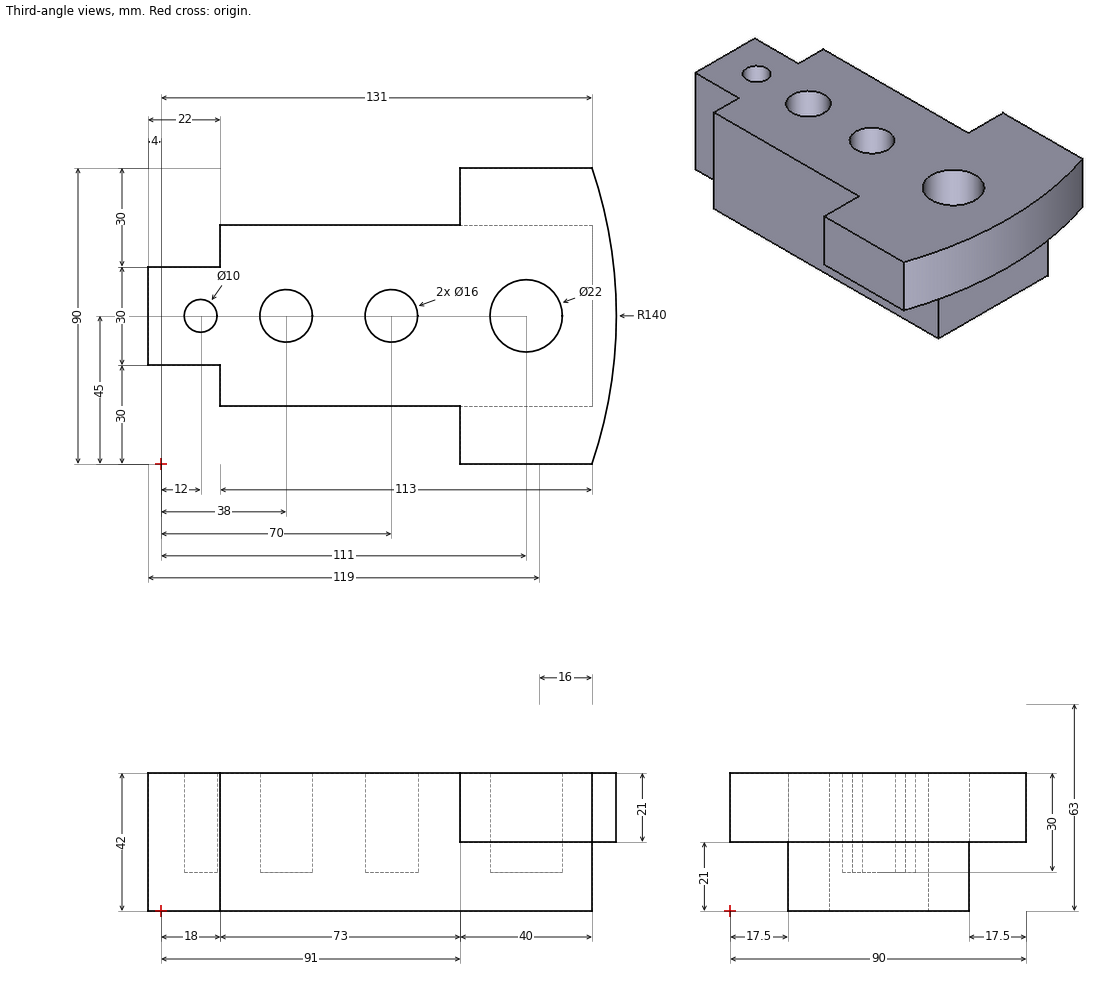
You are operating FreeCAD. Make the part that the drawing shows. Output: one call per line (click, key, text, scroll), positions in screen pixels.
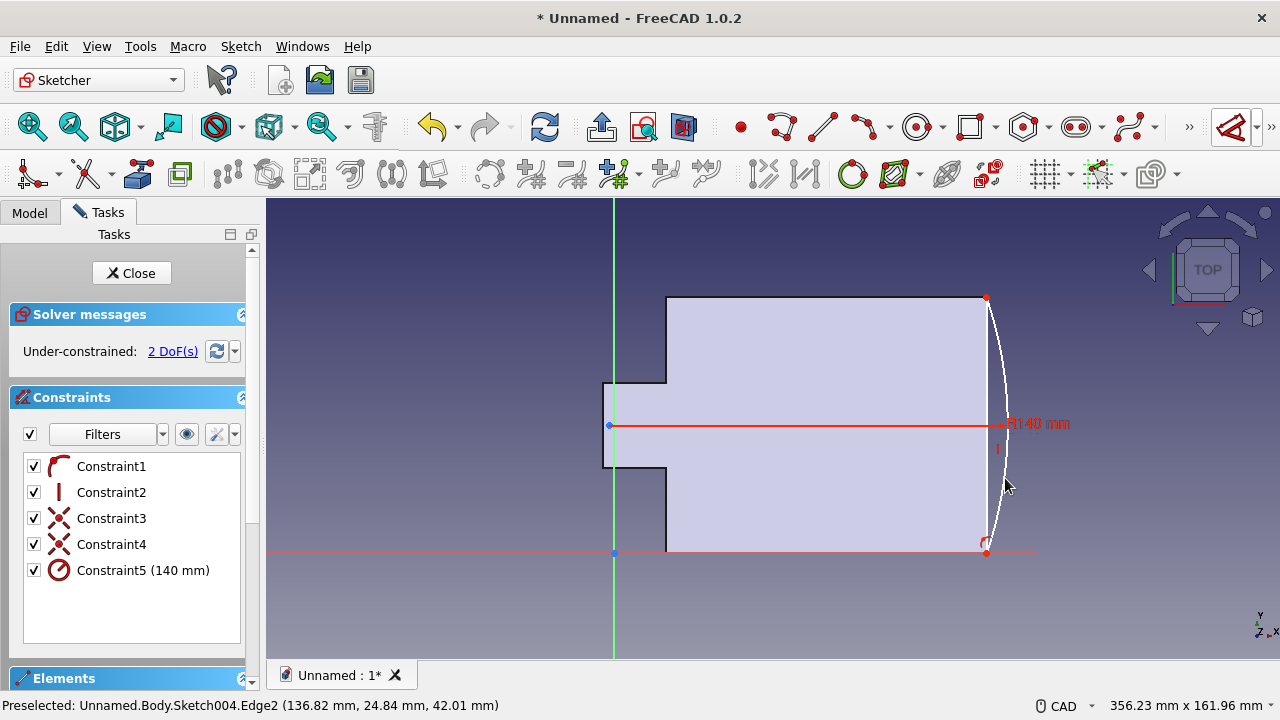
click(987, 375)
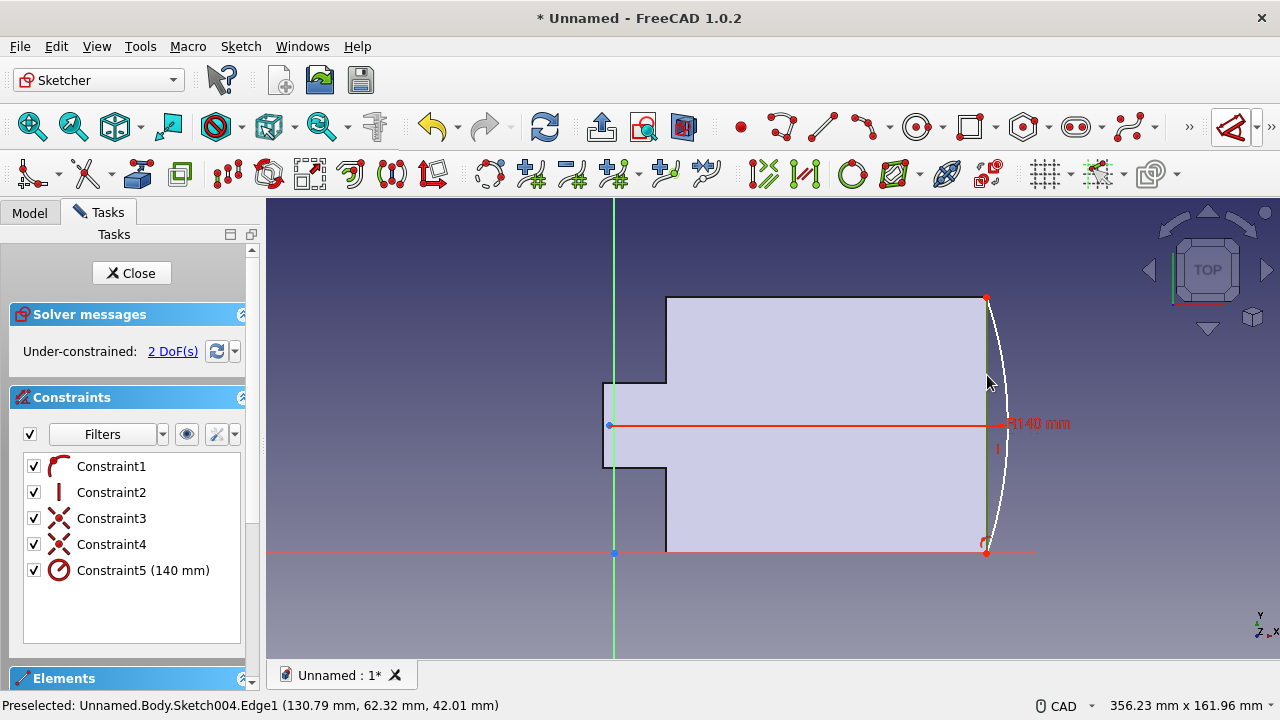
key(i)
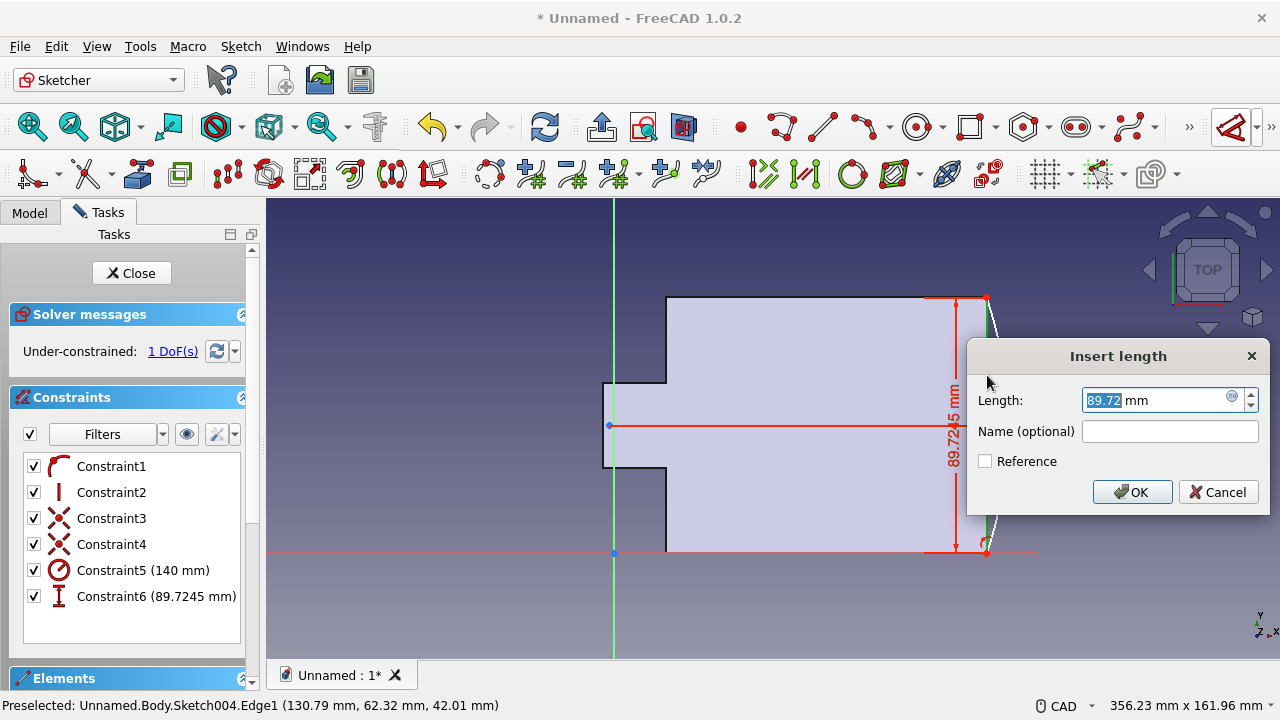
text(90)
key(Return)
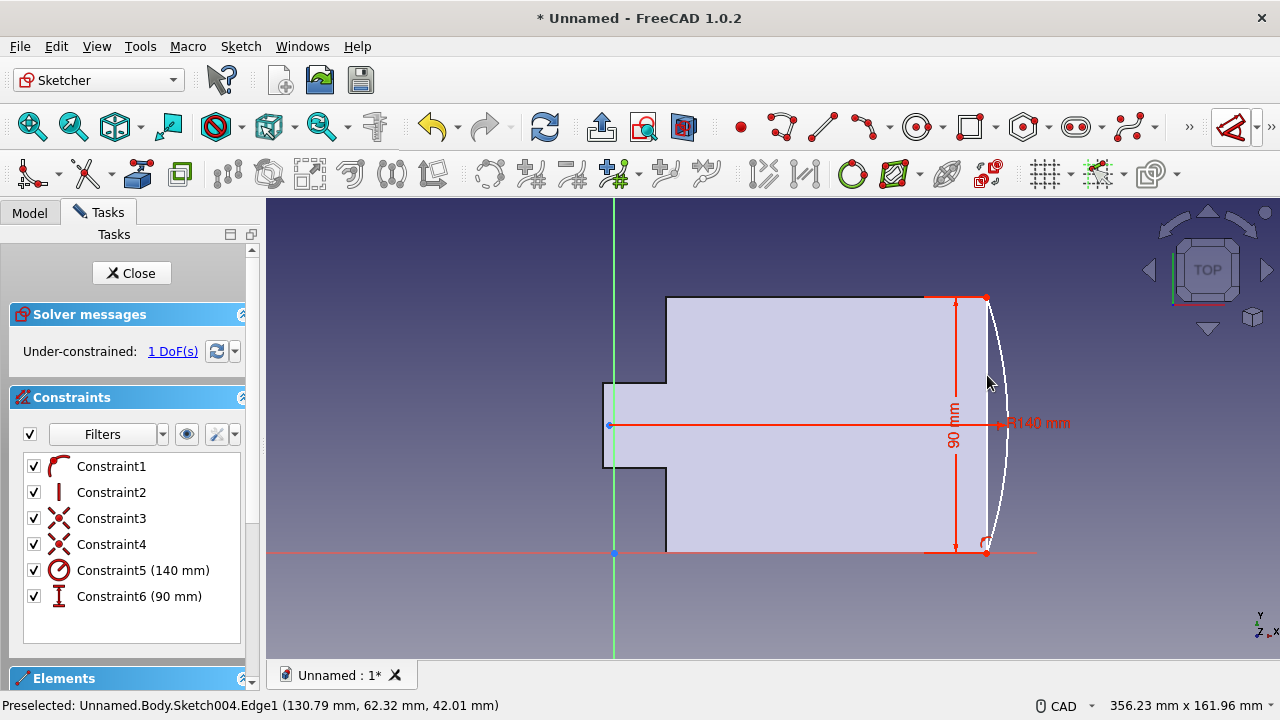
click(987, 297)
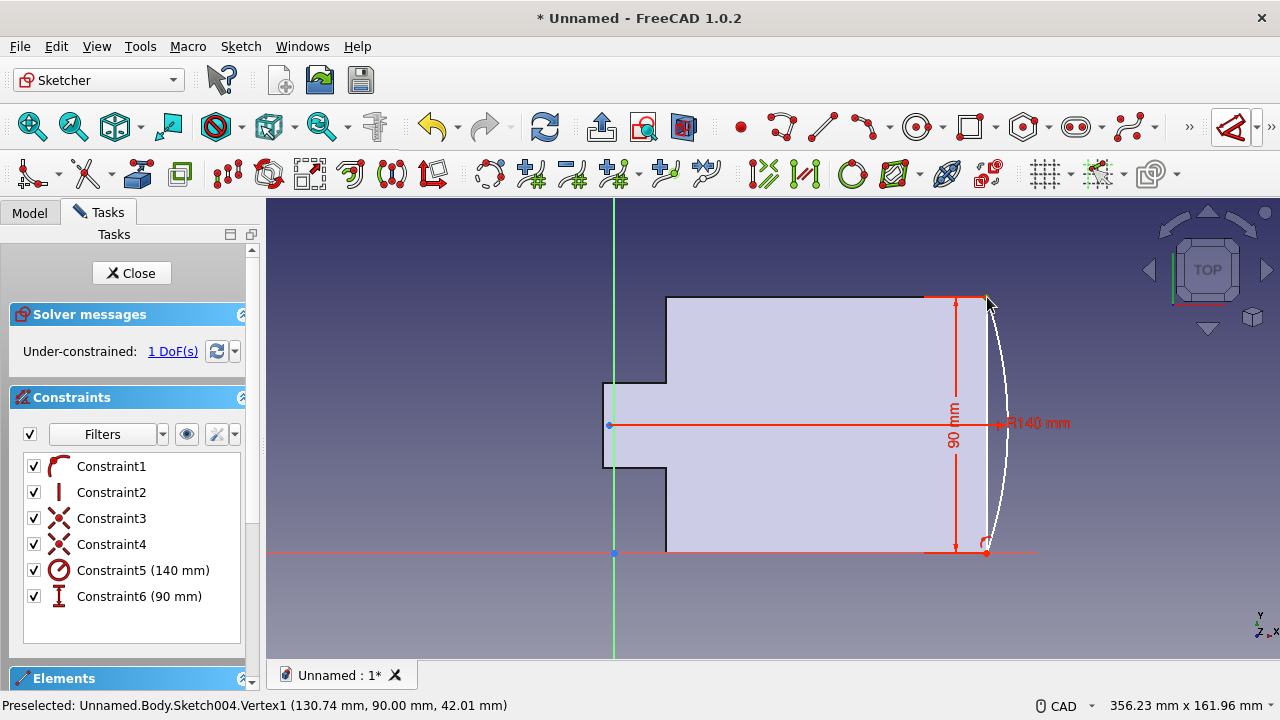
click(1256, 128)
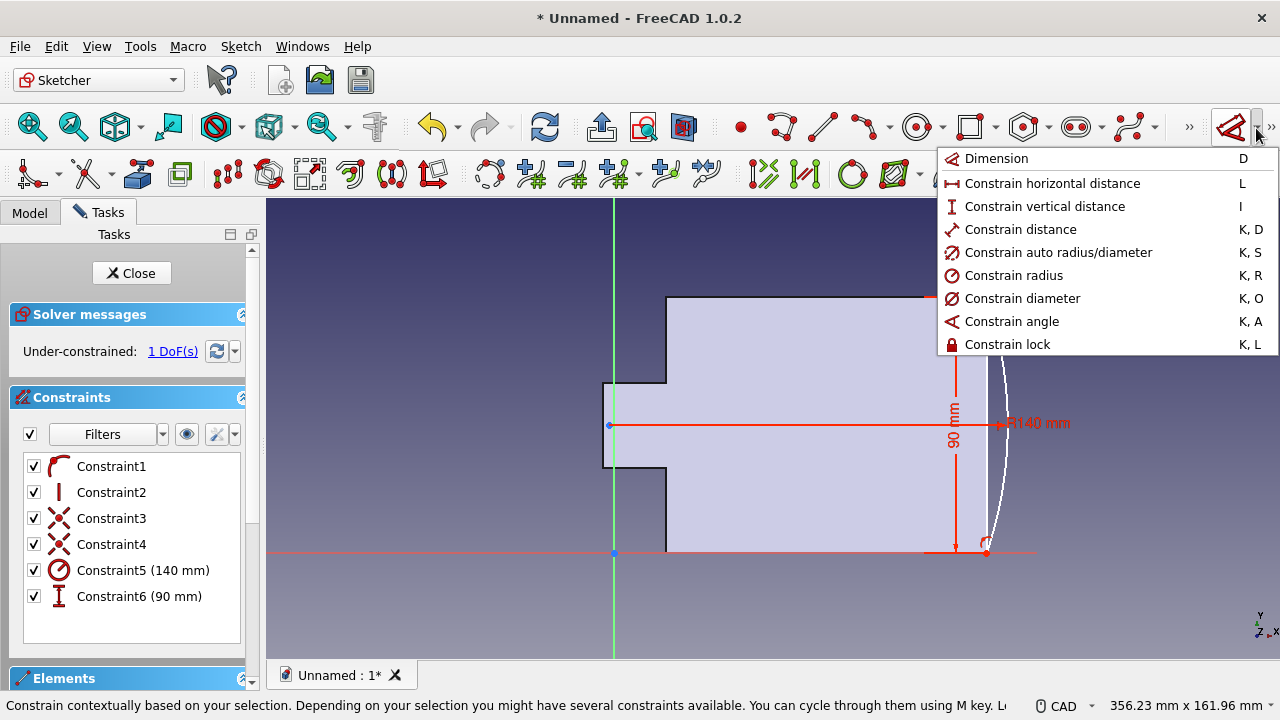
click(1108, 184)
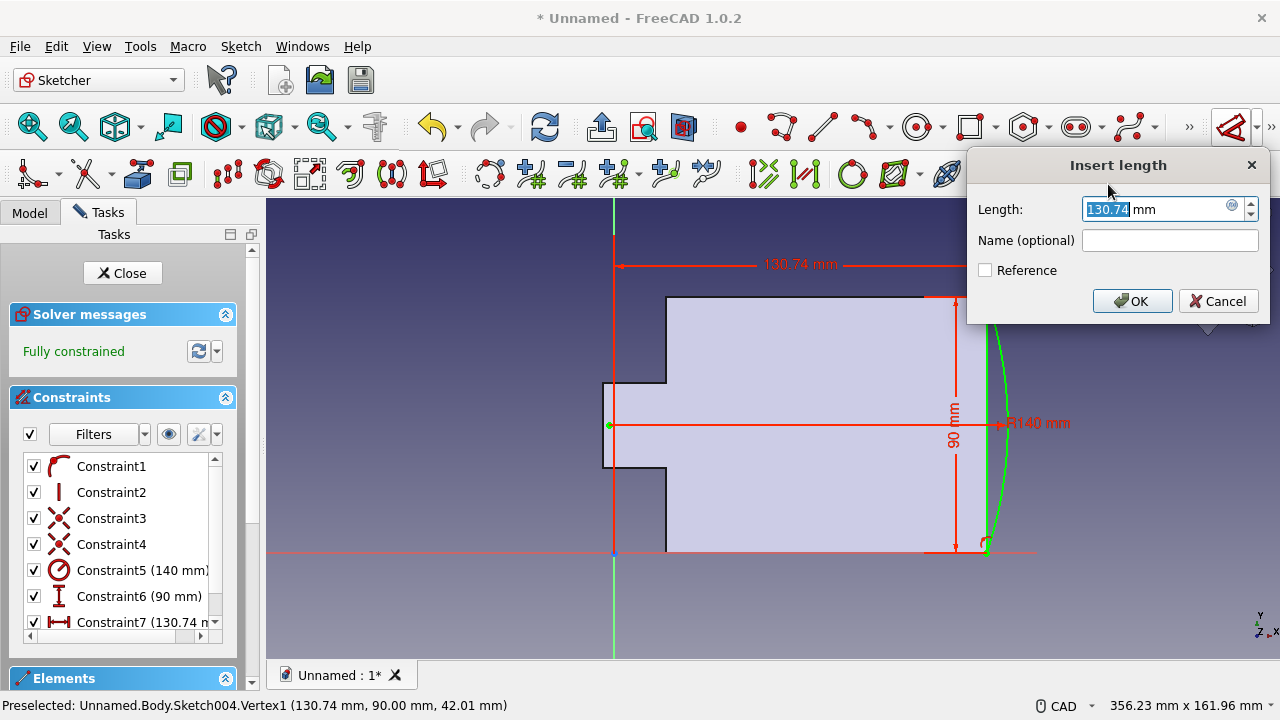
text(131)
key(Return)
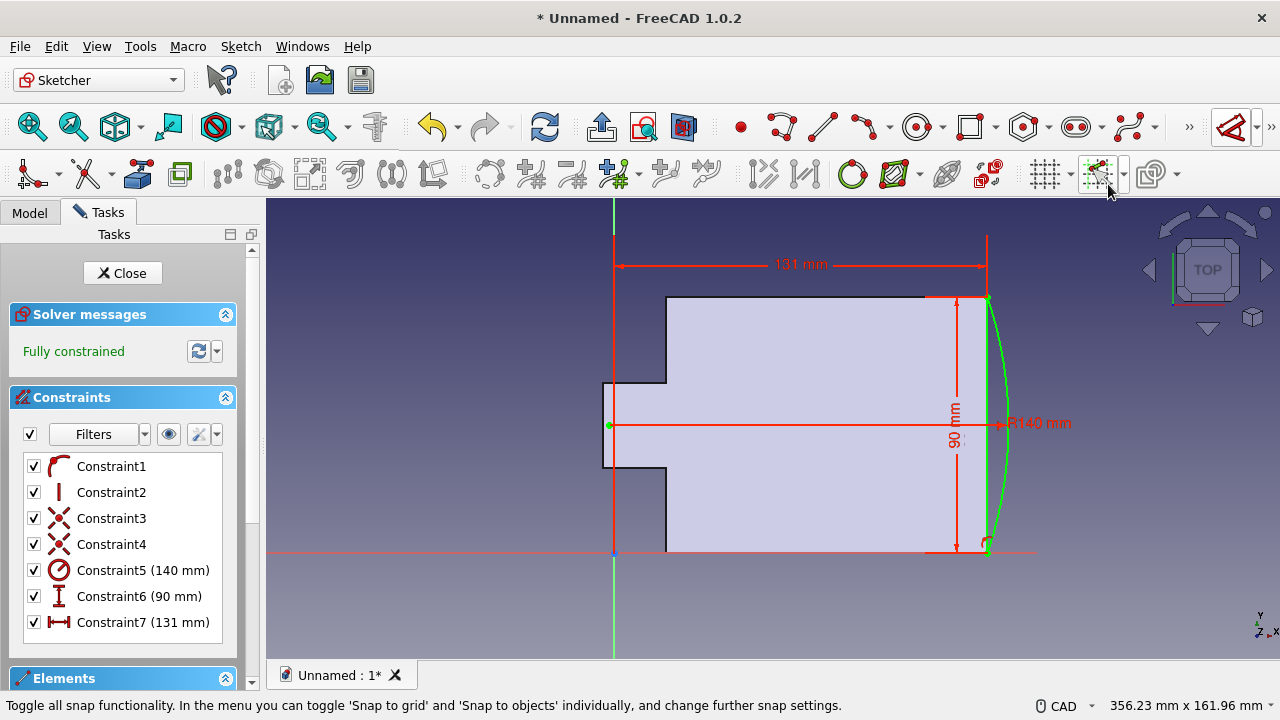
click(123, 273)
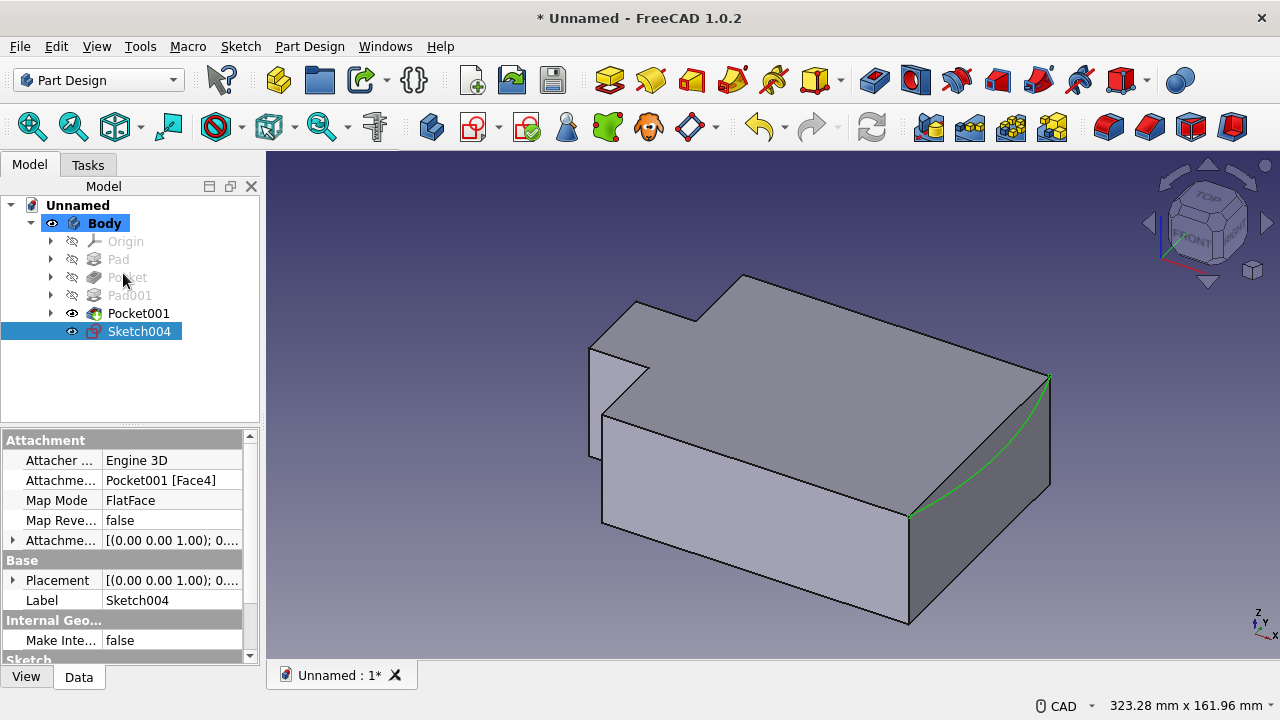
click(610, 80)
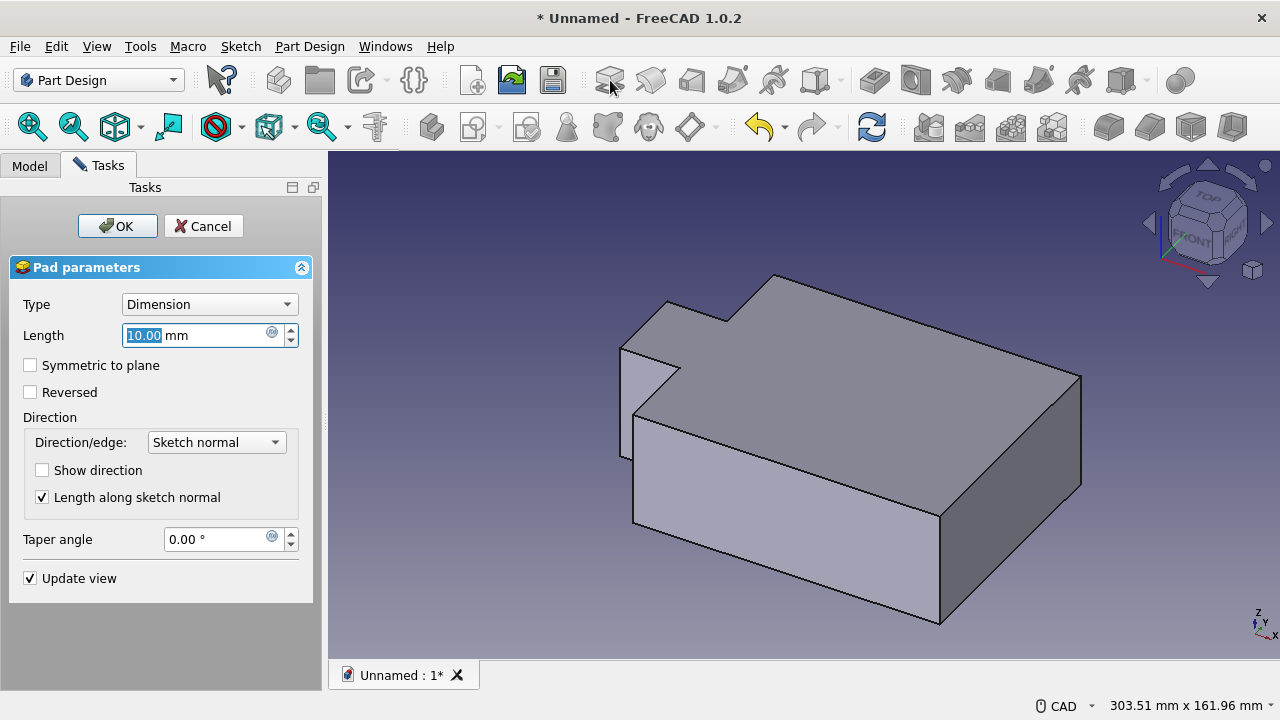
text(21)
key(Tab)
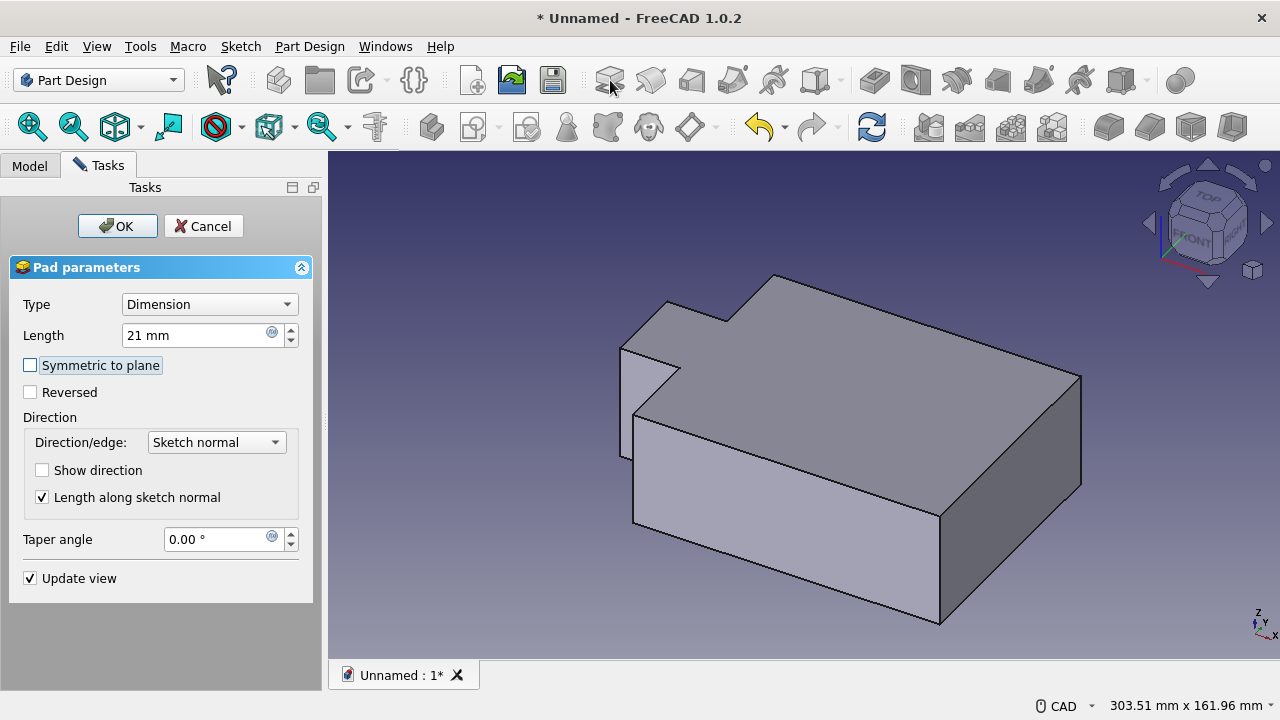
click(31, 392)